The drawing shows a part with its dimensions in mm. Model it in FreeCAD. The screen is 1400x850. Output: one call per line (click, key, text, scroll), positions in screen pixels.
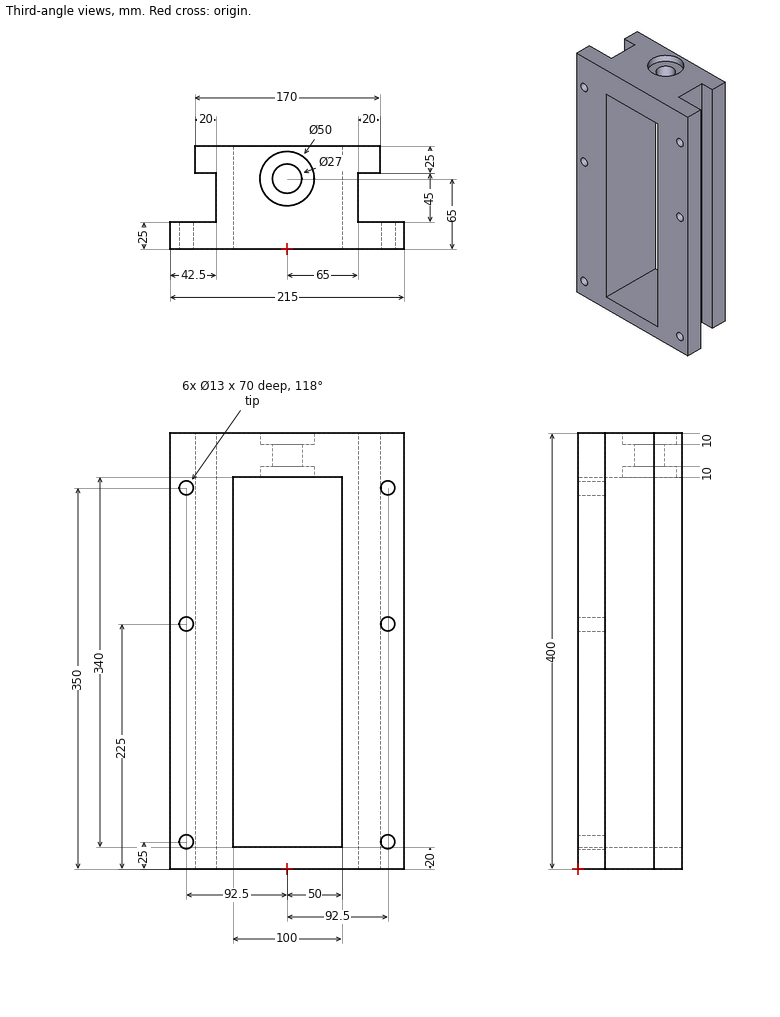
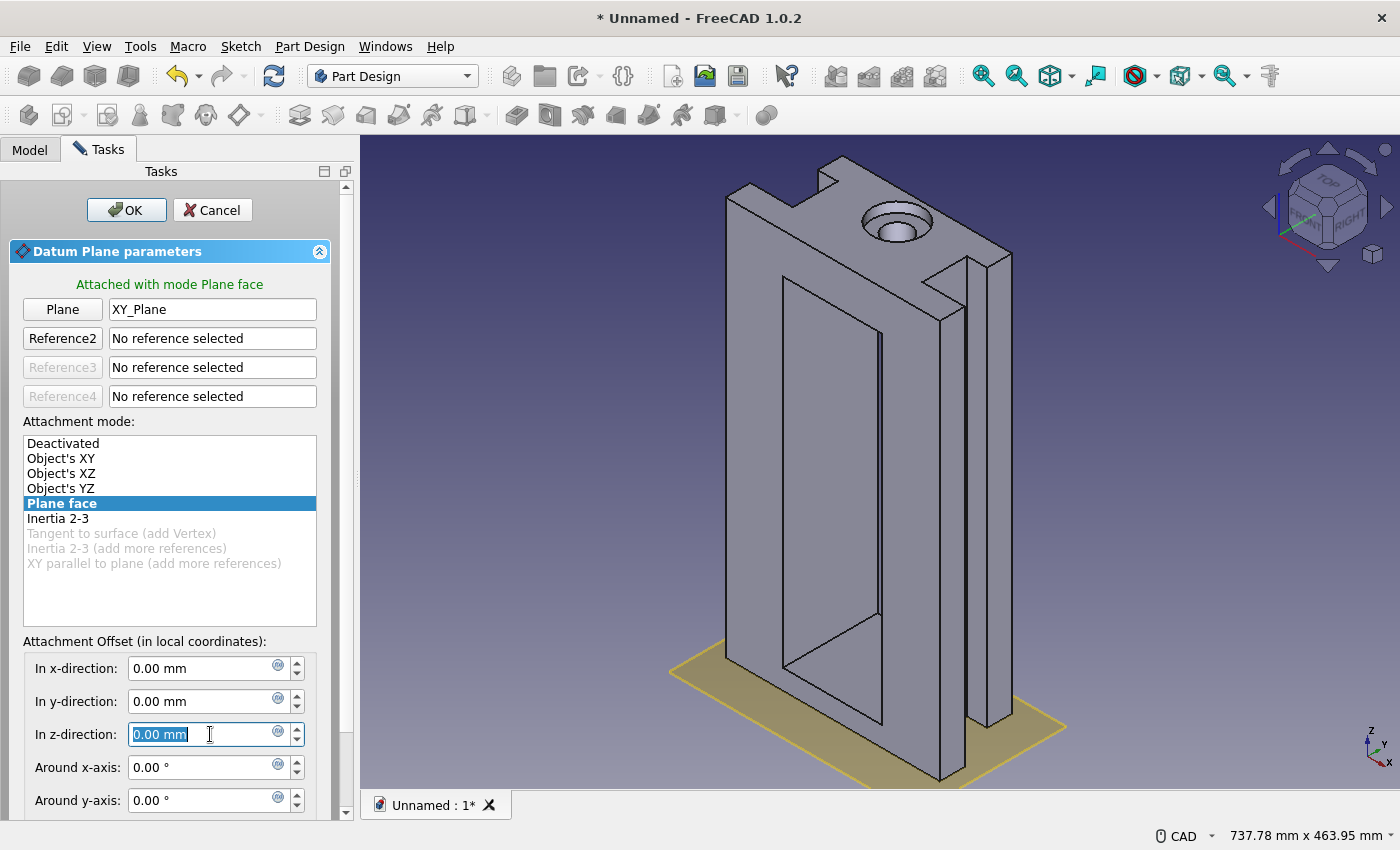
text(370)
key(Tab)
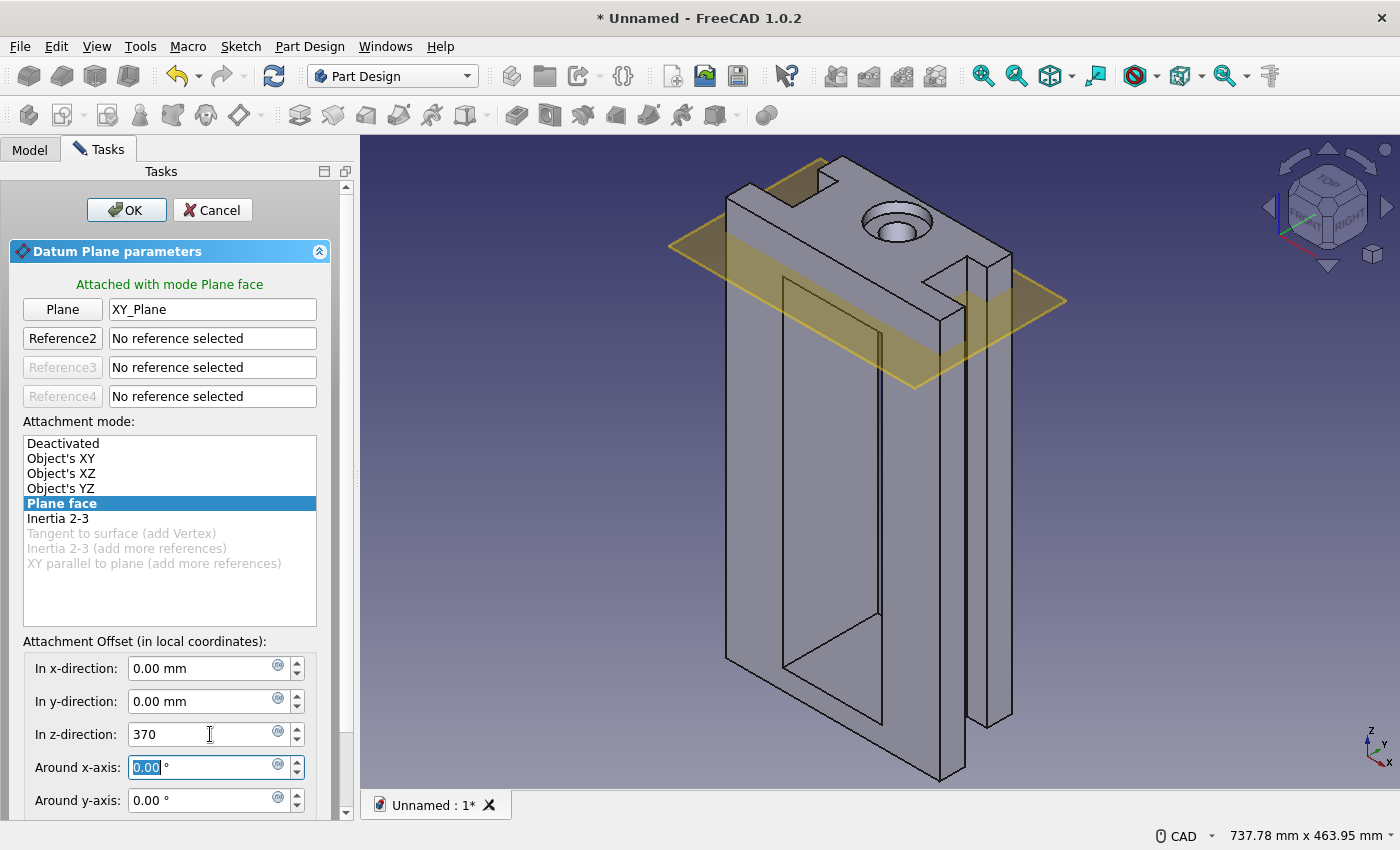
click(127, 210)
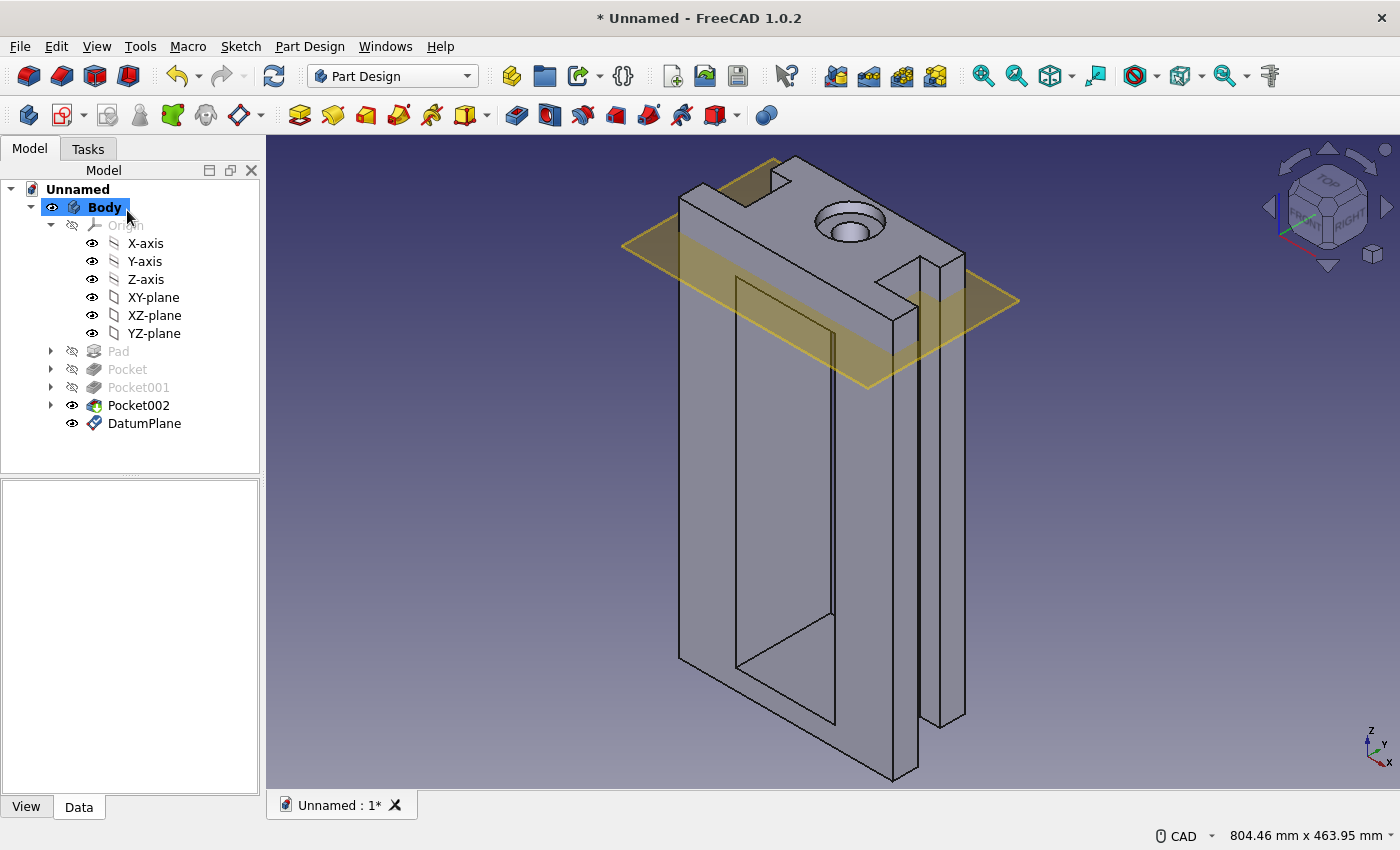
click(117, 423)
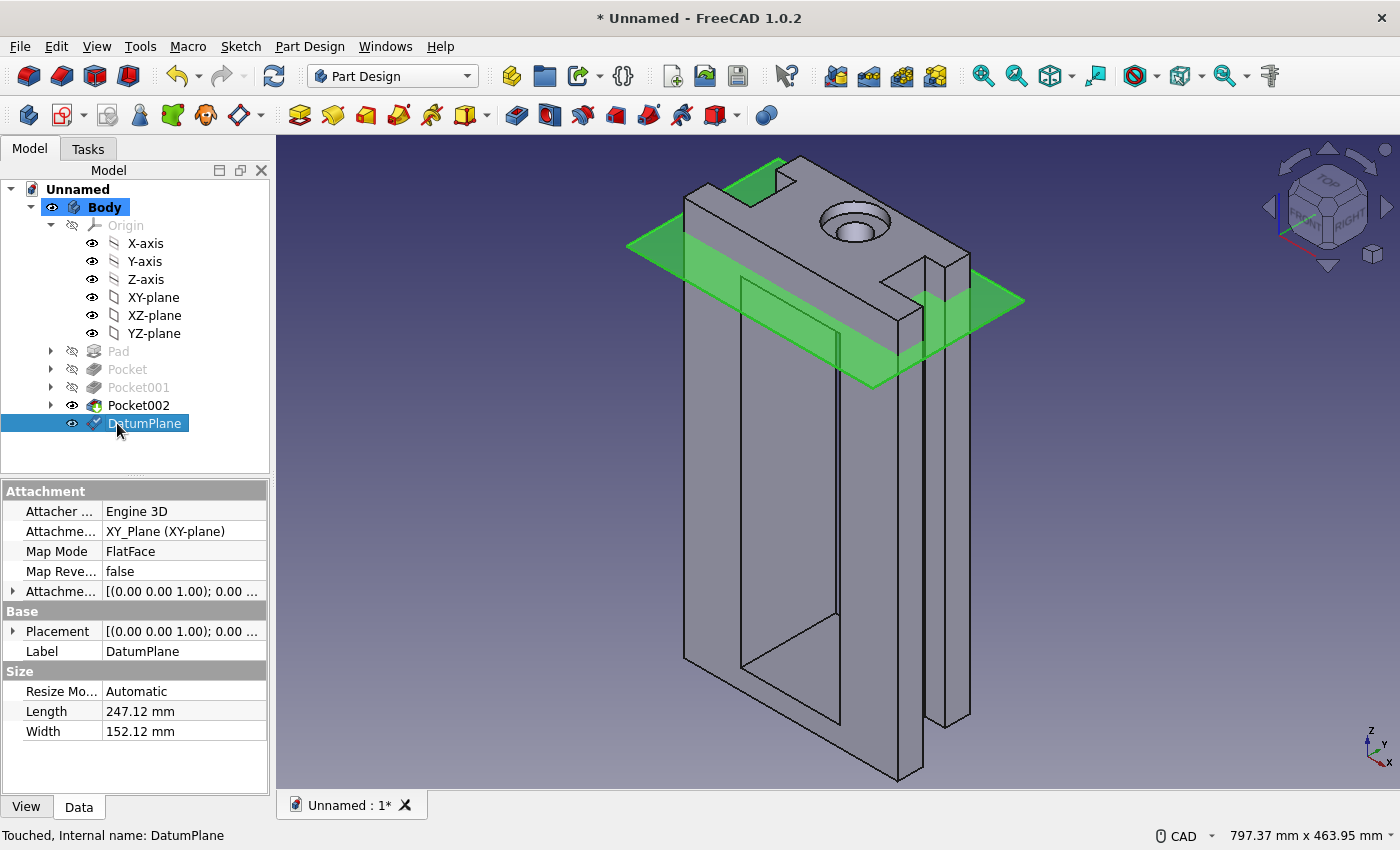
click(62, 116)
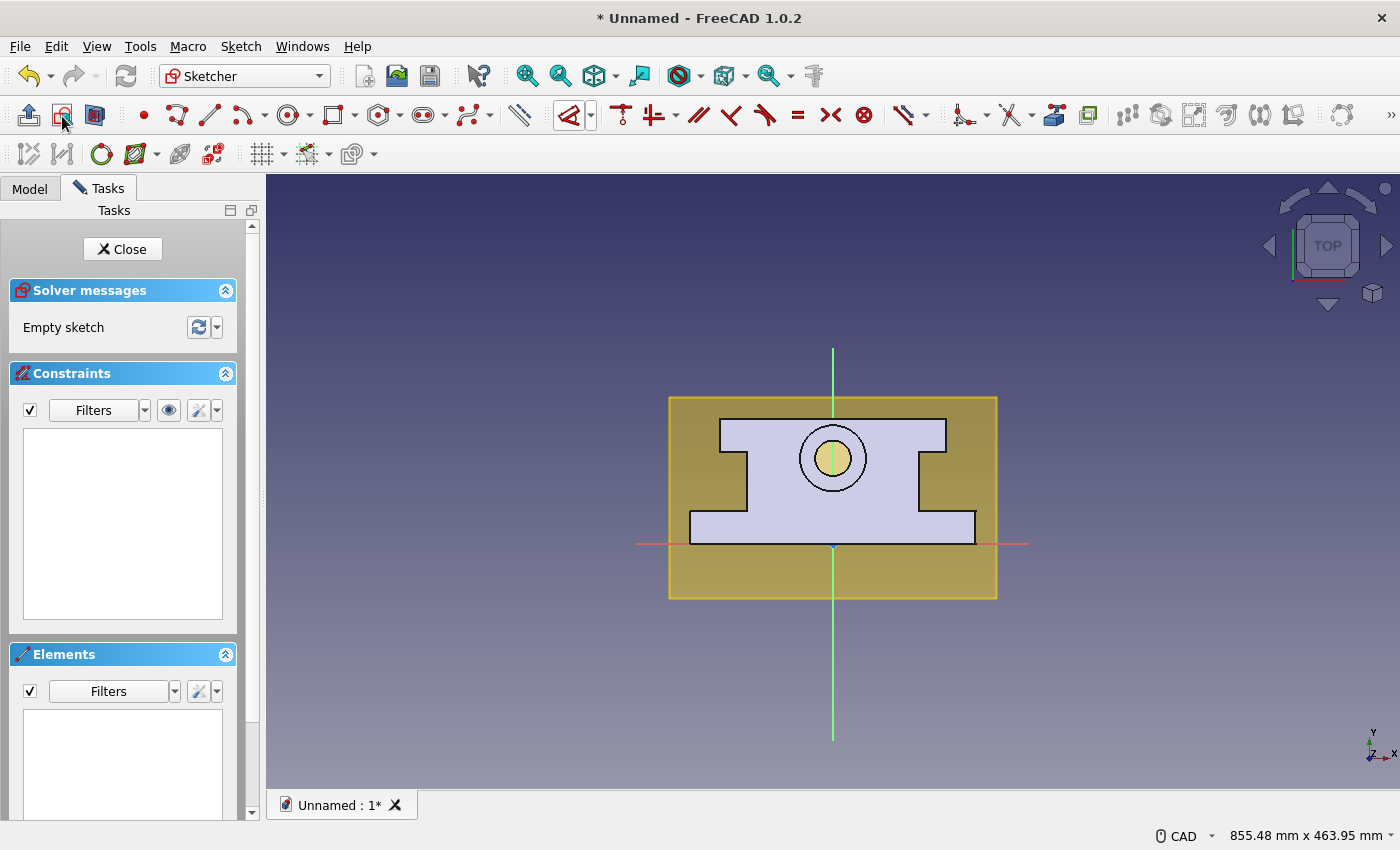
key(q)
key(s)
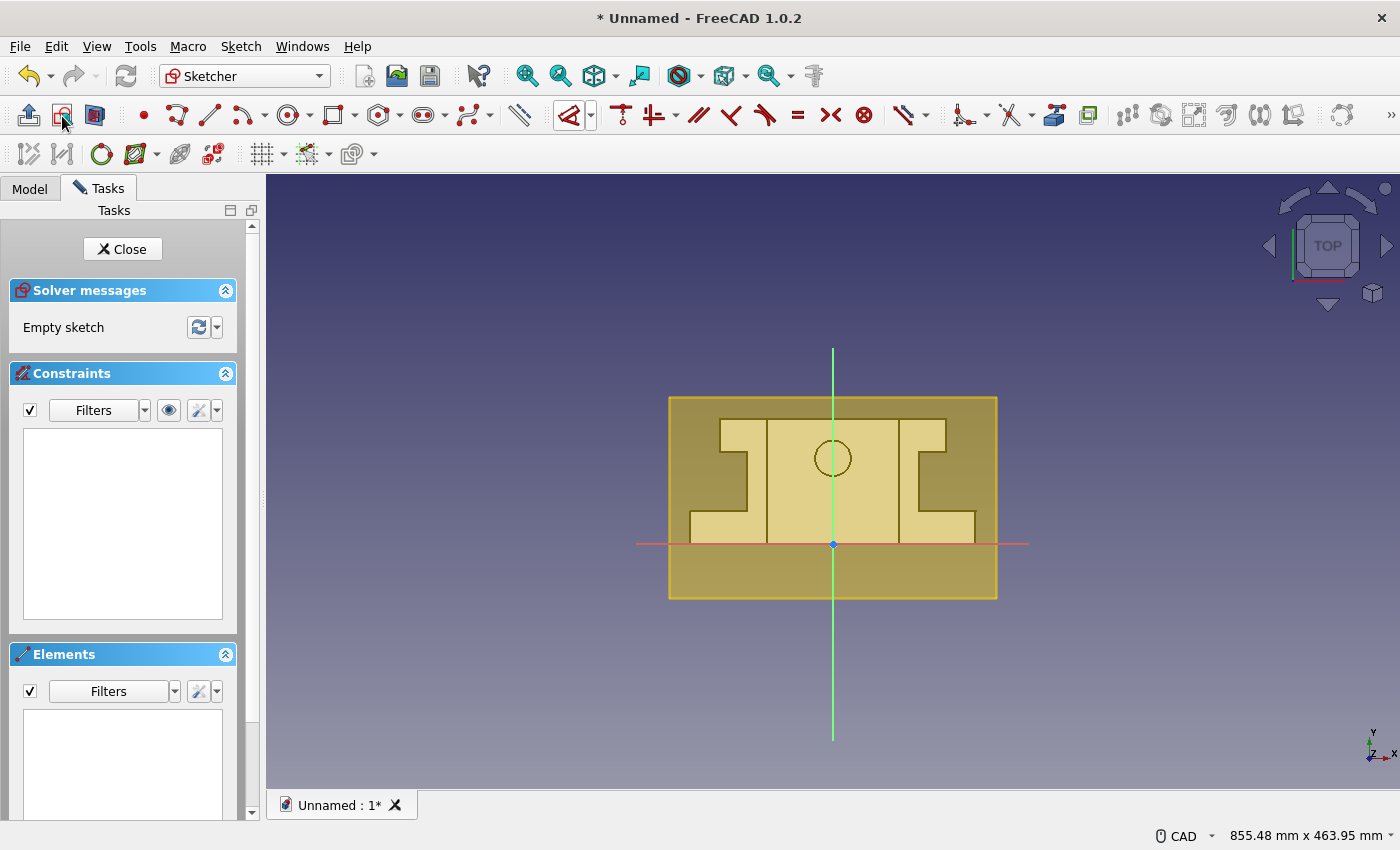
scroll(863, 486, up, 6)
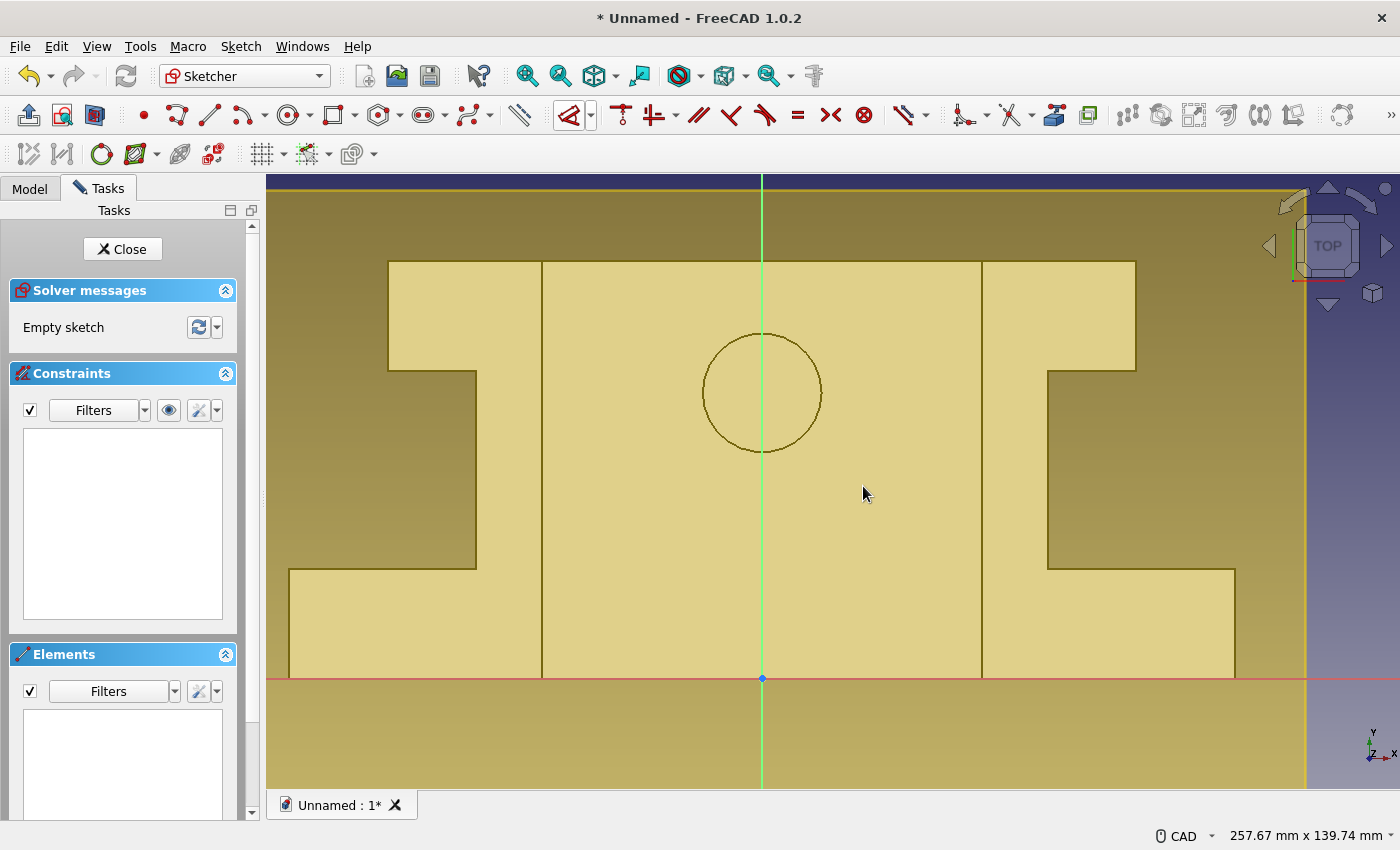
click(288, 116)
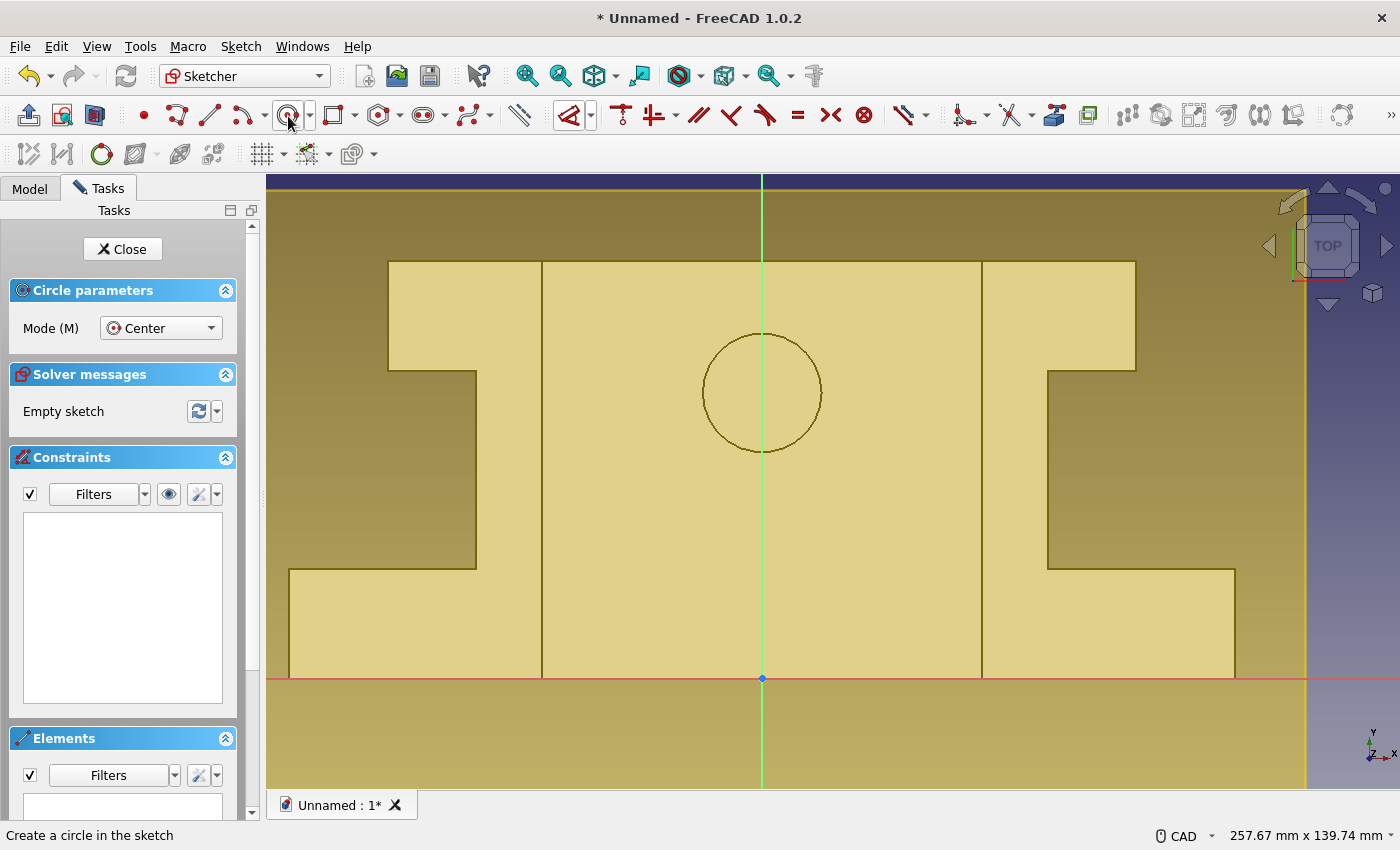
click(762, 393)
move(840, 315)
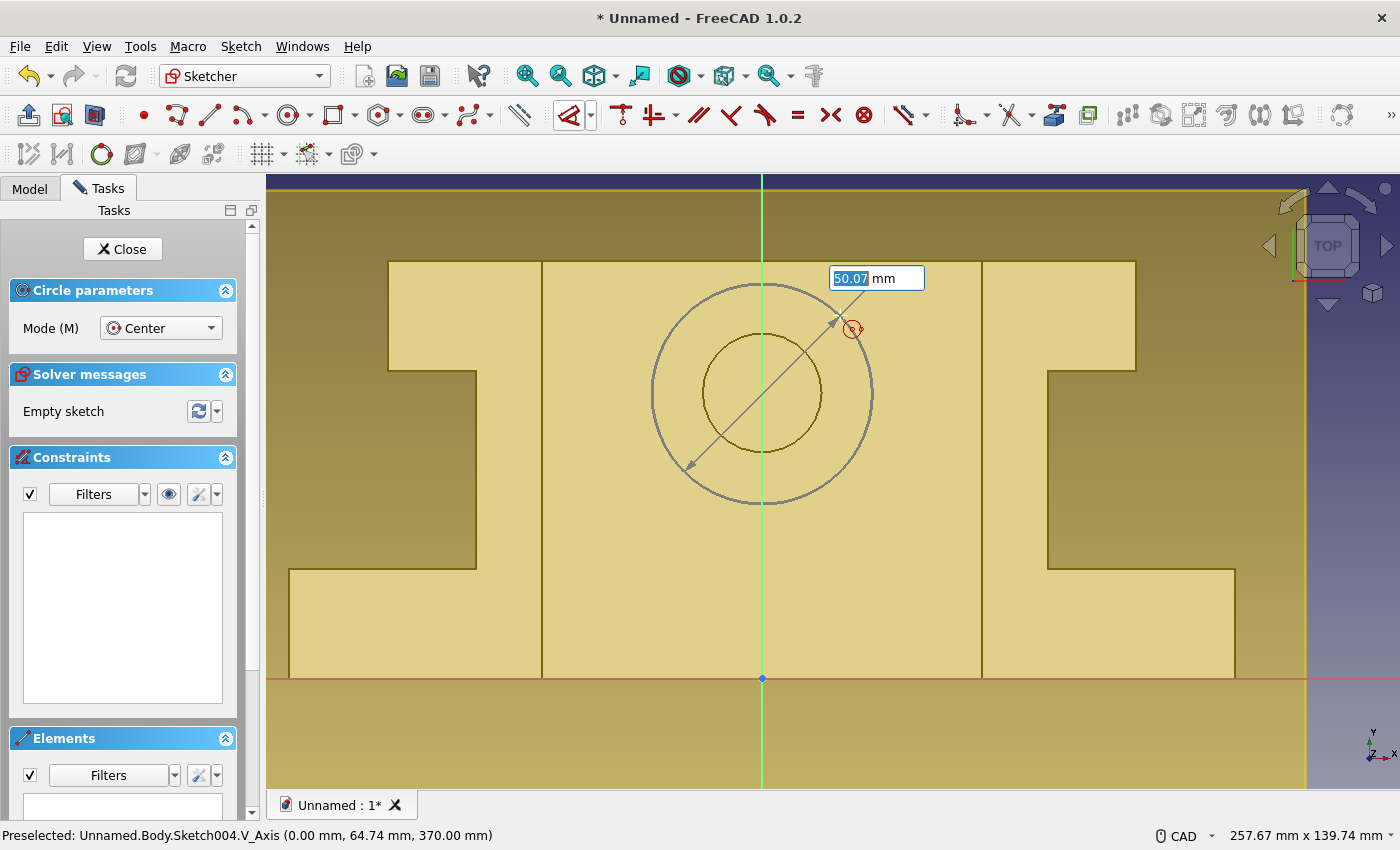
text(50)
key(Return)
key(Escape)